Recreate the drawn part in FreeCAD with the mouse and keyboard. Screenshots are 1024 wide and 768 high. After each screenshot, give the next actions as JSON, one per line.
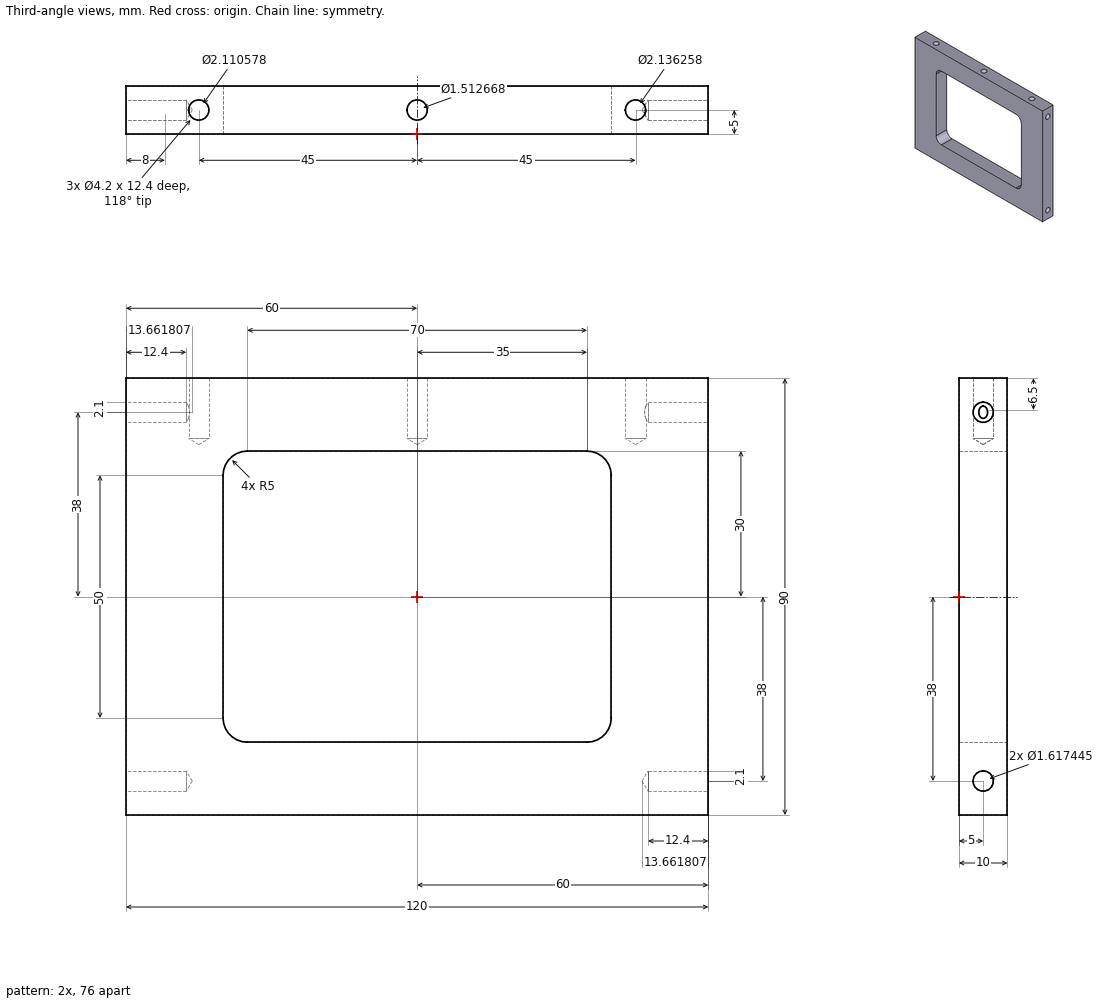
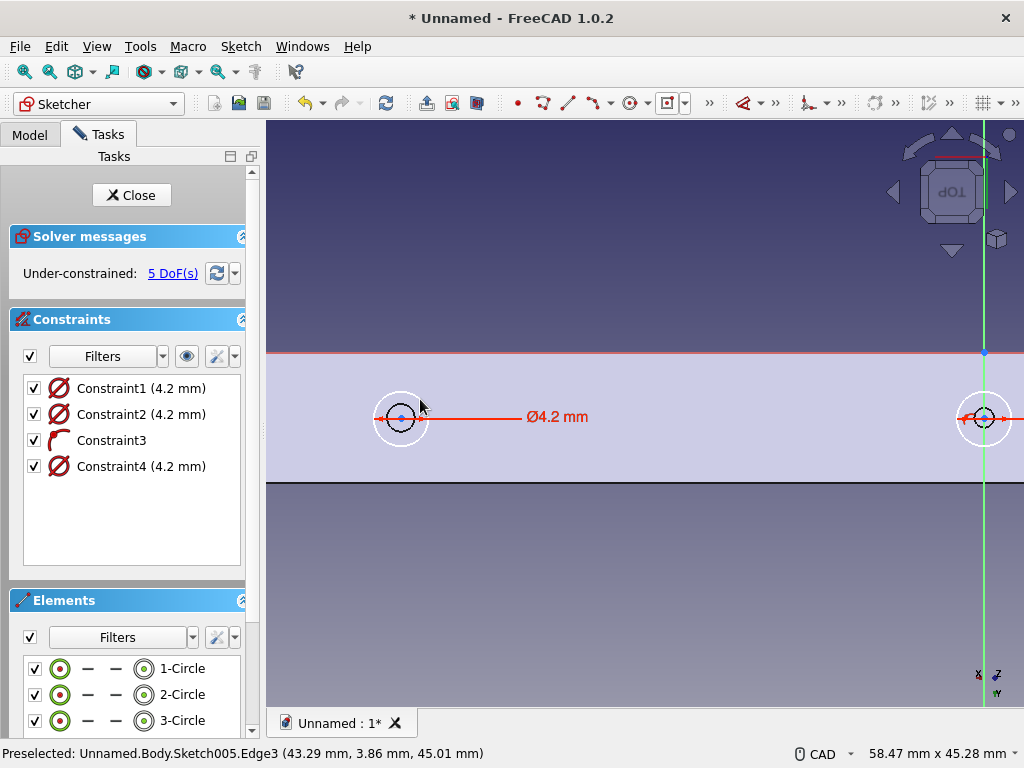
{"action": "scroll", "coordinate": [401, 420], "scroll_direction": "down", "scroll_amount": 6}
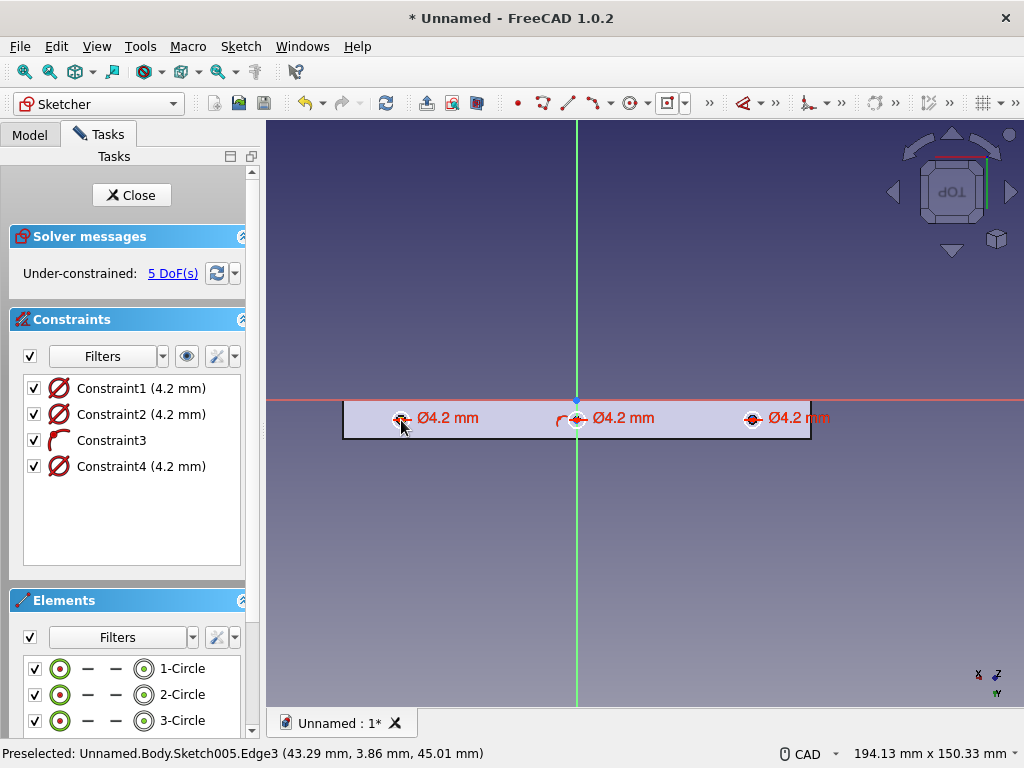
{"action": "left_click", "coordinate": [753, 420]}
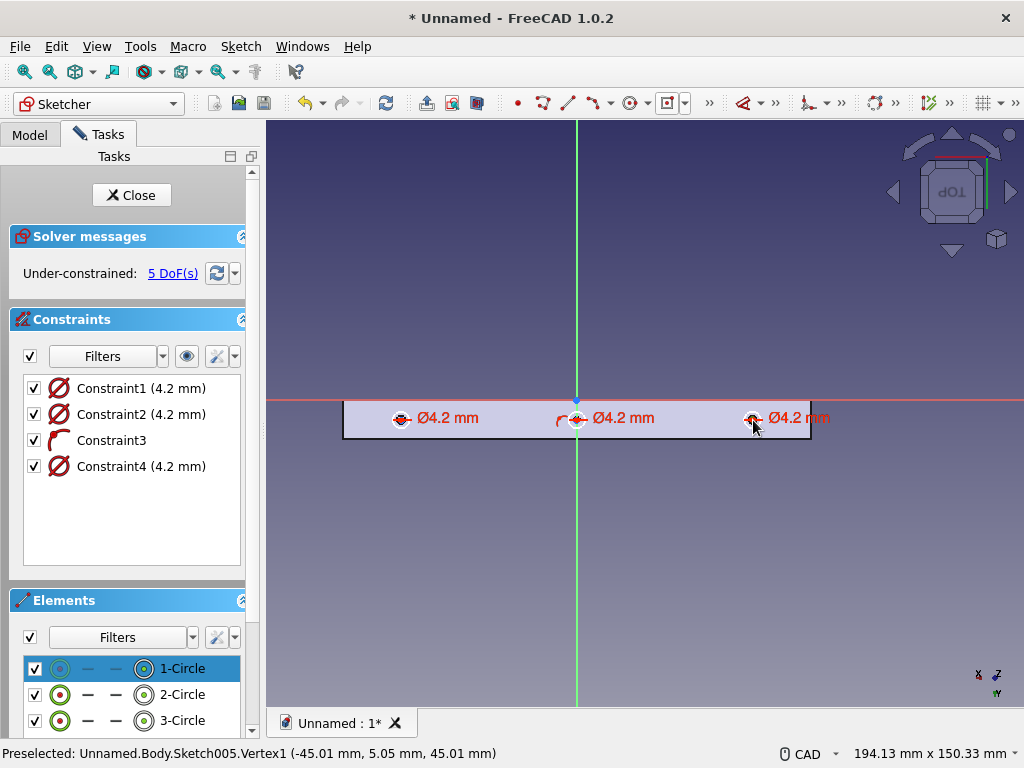
{"action": "left_click", "coordinate": [401, 420]}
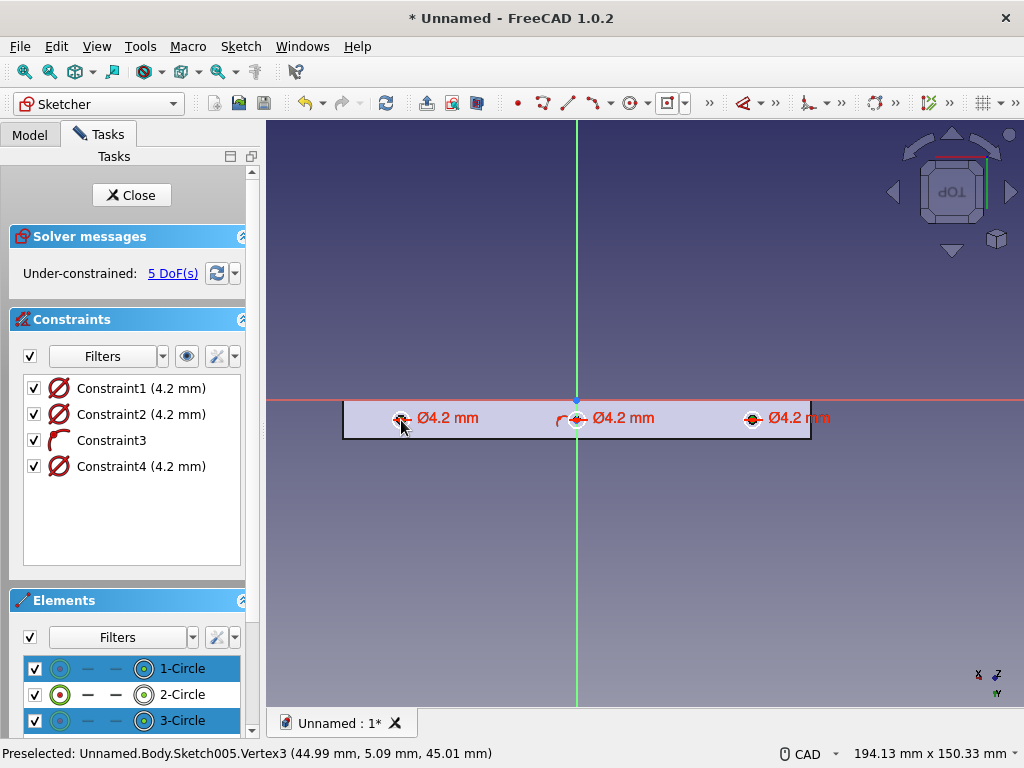
{"action": "left_click", "coordinate": [577, 641]}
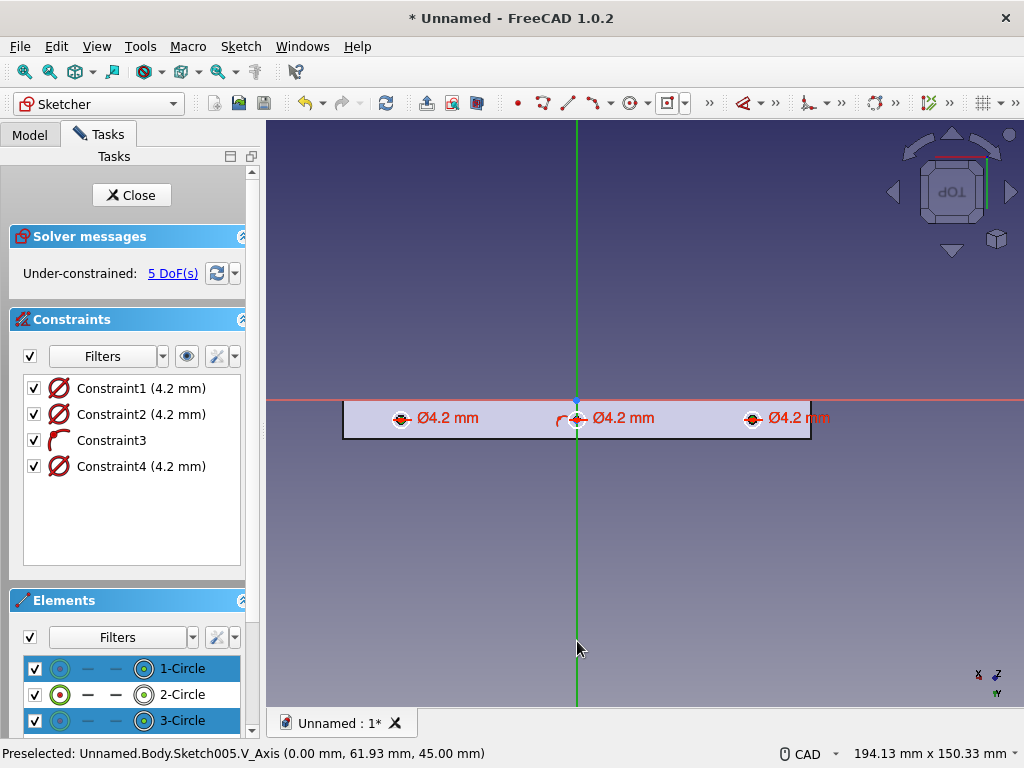
{"action": "key", "text": "s"}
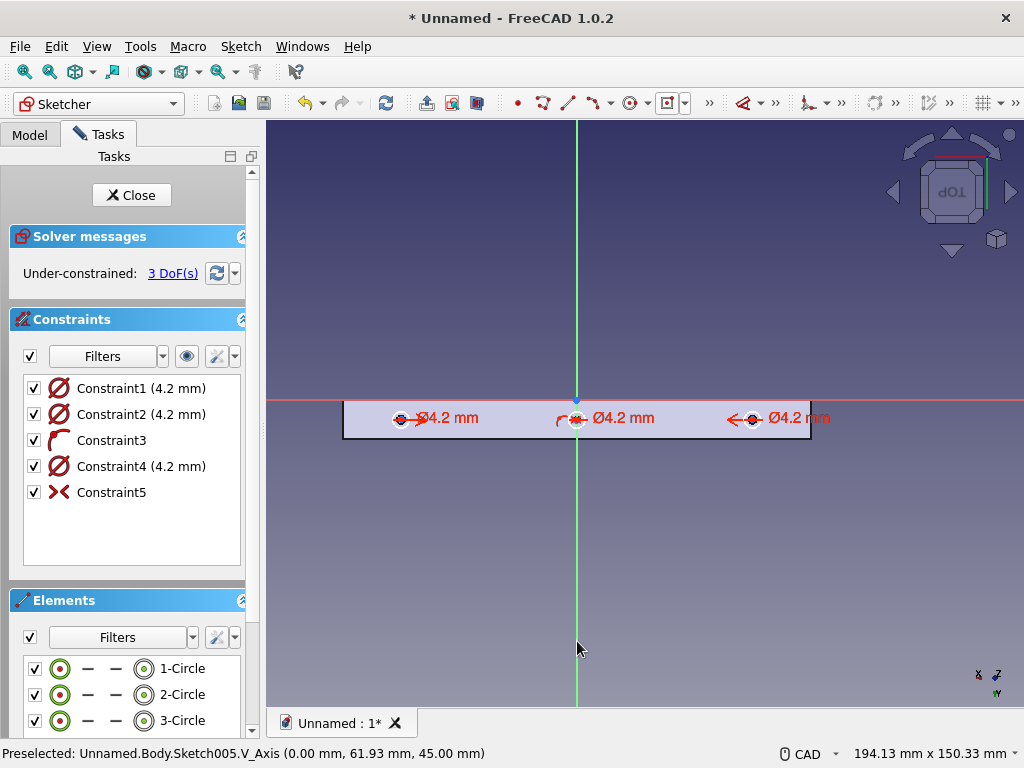
{"action": "left_click", "coordinate": [742, 104]}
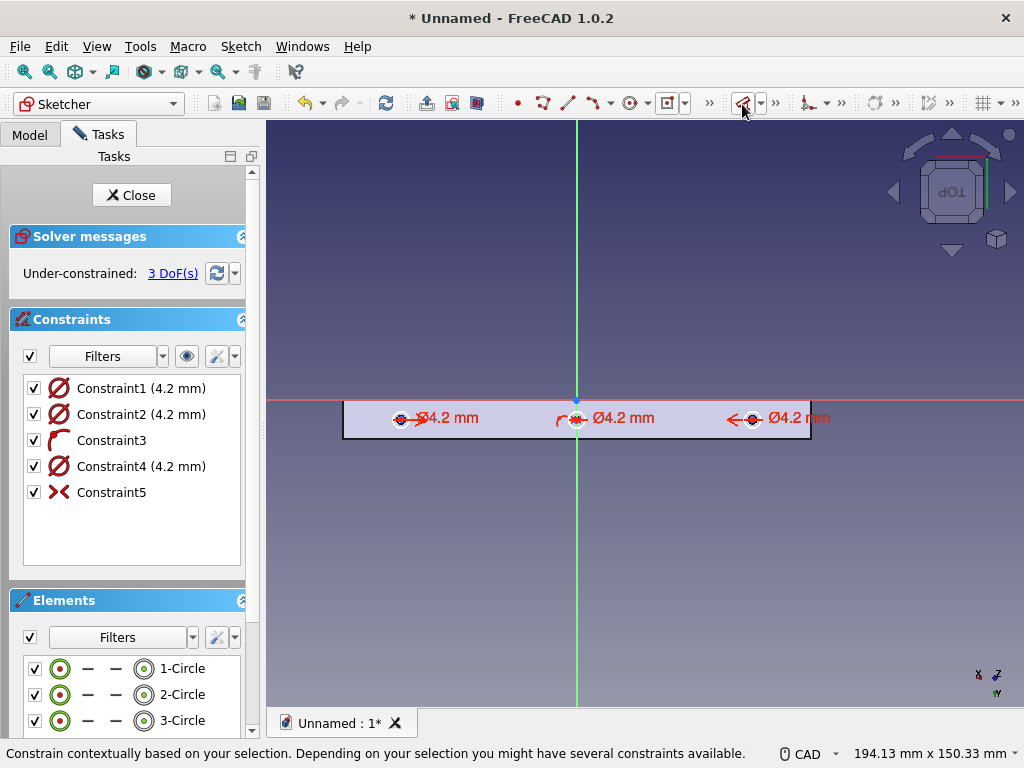
{"action": "scroll", "coordinate": [753, 420], "scroll_direction": "up", "scroll_amount": 4}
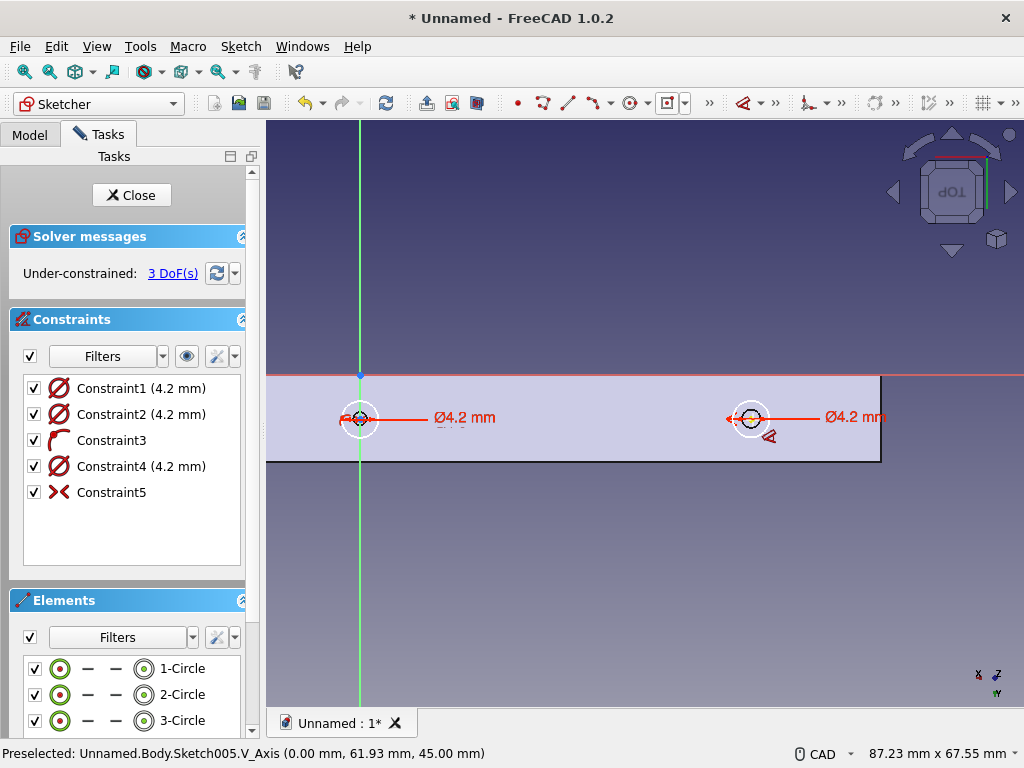
{"action": "left_click", "coordinate": [751, 419]}
{"action": "left_click", "coordinate": [785, 397]}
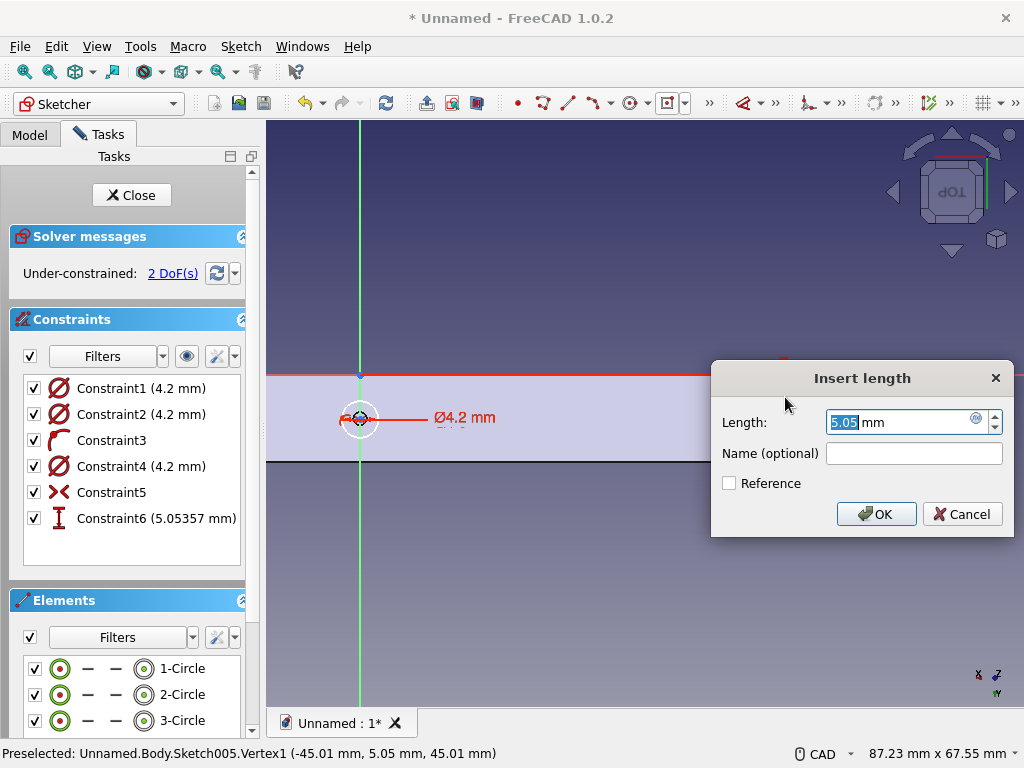
{"action": "type", "text": "5"}
{"action": "key", "text": "Return"}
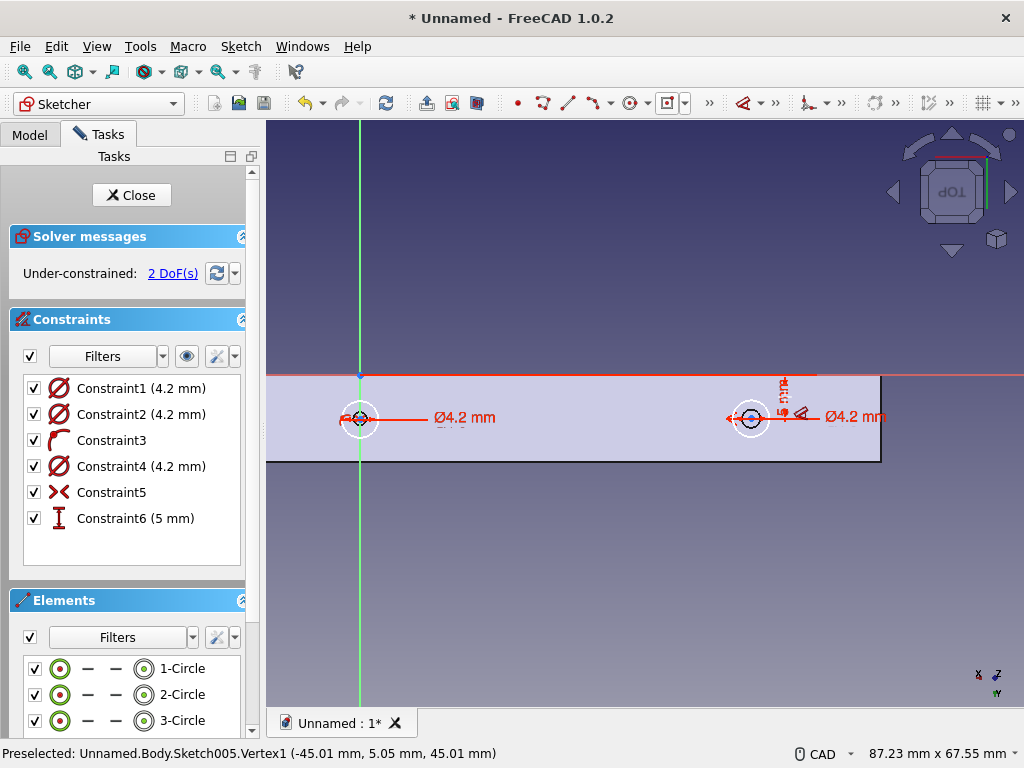
{"action": "left_click", "coordinate": [360, 419]}
{"action": "left_click", "coordinate": [394, 397]}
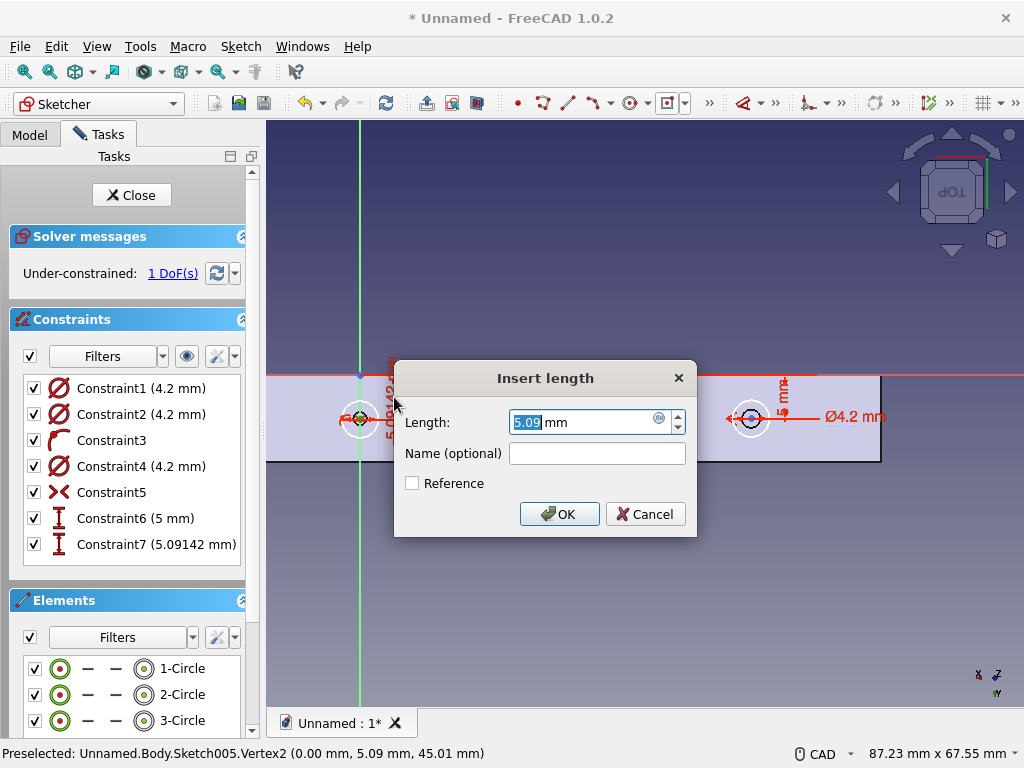
{"action": "type", "text": "5"}
{"action": "key", "text": "Return"}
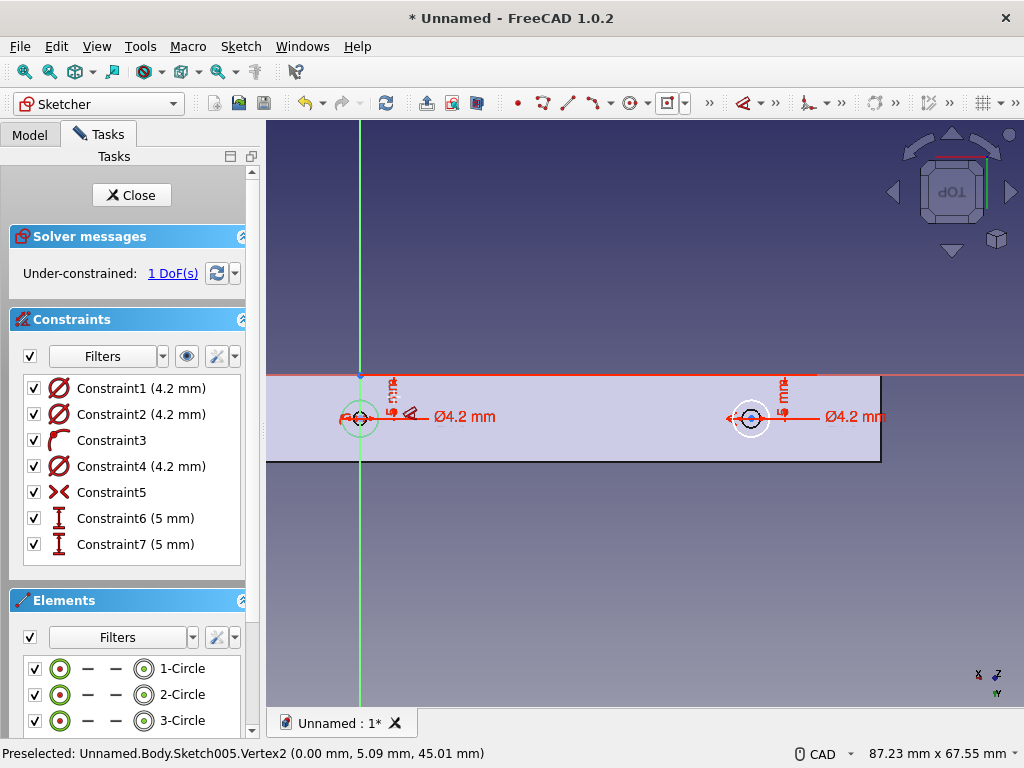
{"action": "left_click", "coordinate": [751, 419]}
{"action": "left_click", "coordinate": [556, 341]}